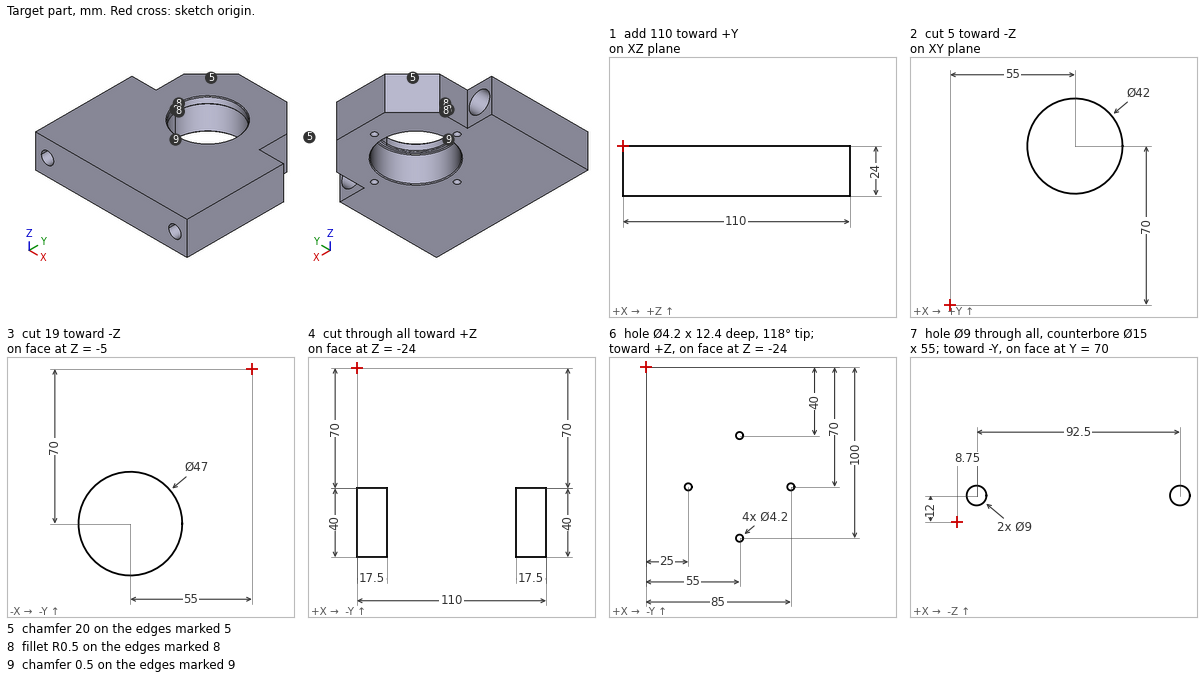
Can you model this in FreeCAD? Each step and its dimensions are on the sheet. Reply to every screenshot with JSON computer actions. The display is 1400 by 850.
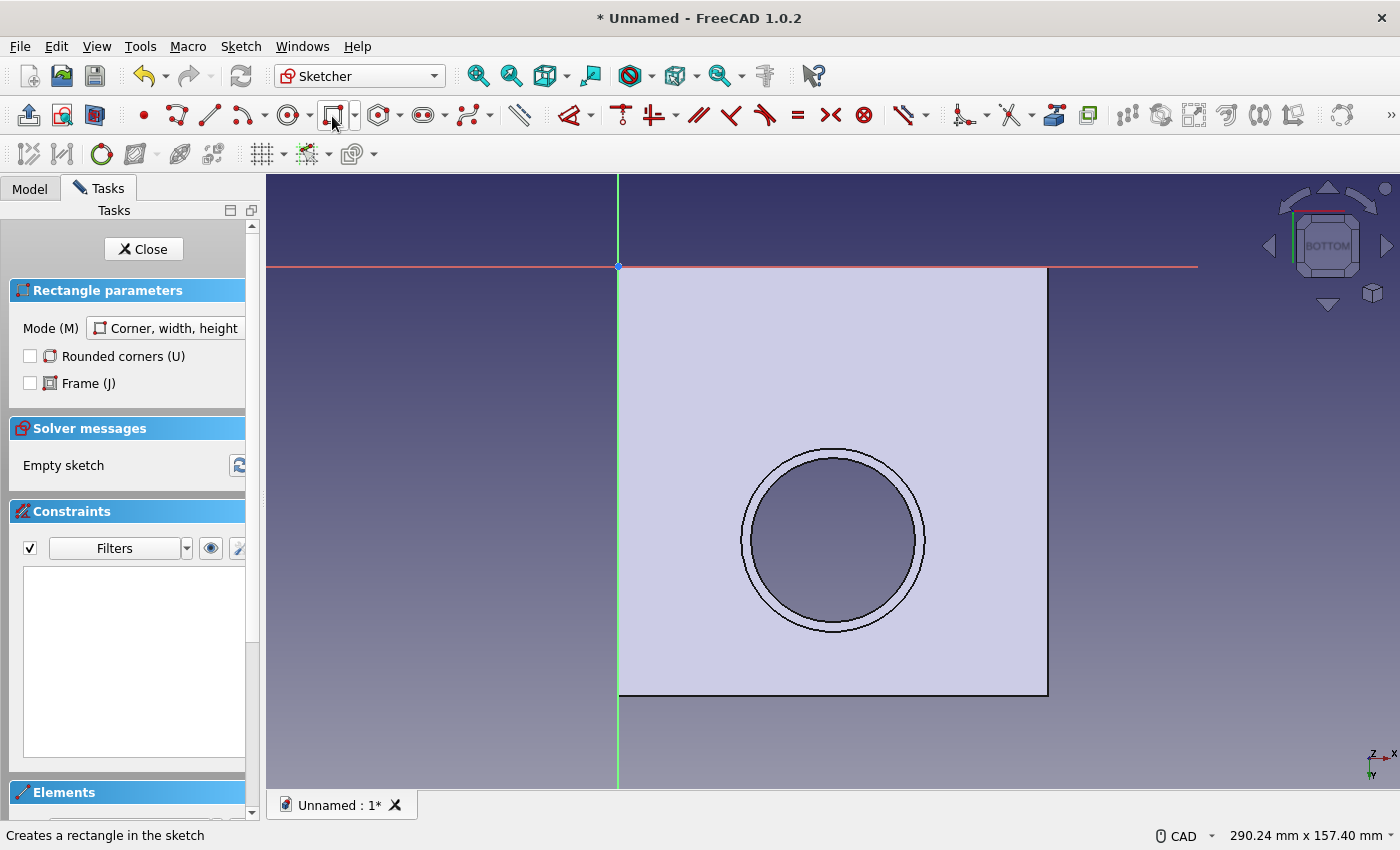
{"action": "left_click", "coordinate": [980, 540]}
{"action": "mouse_move", "coordinate": [1048, 696]}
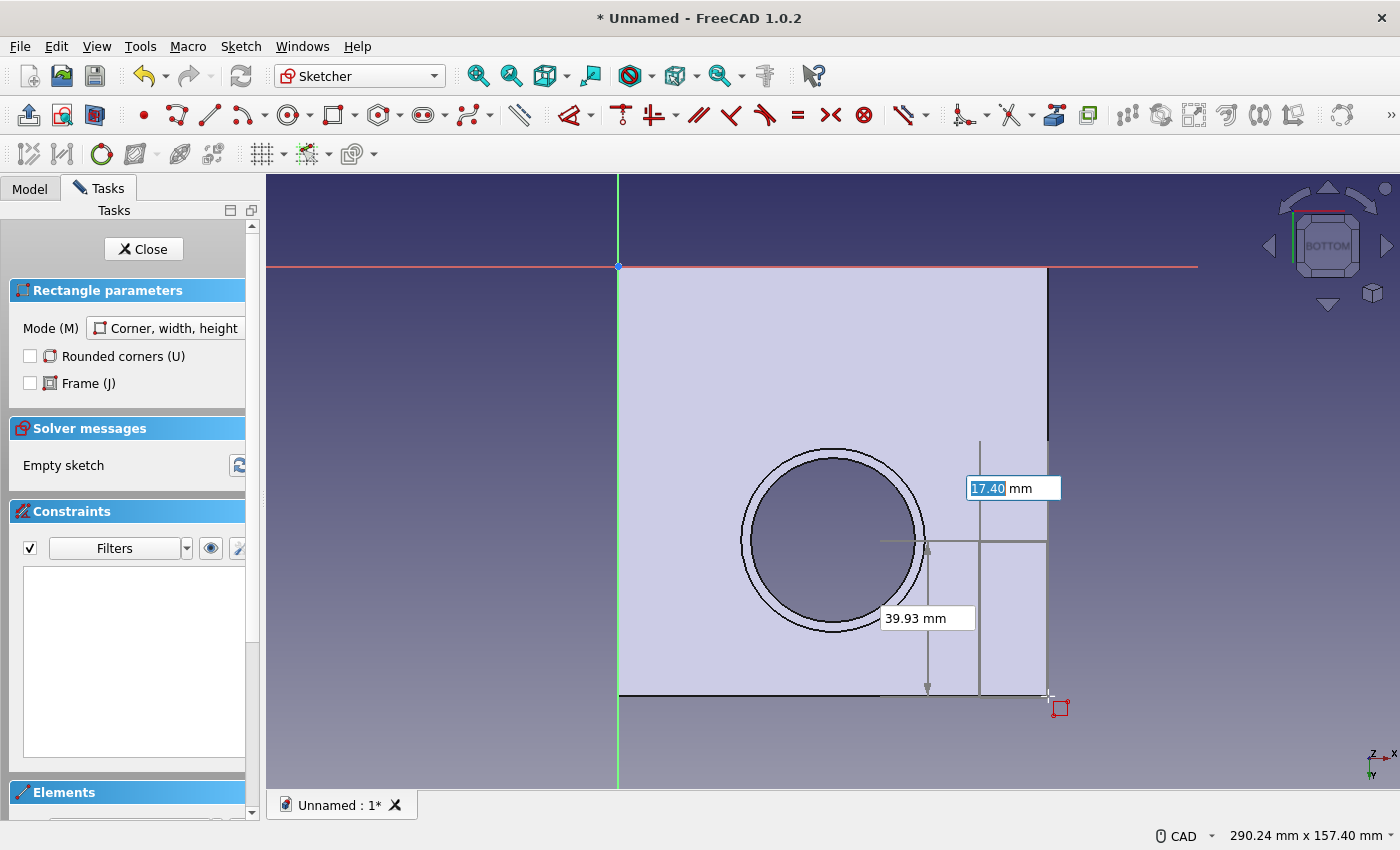
{"action": "type", "text": "17.5"}
{"action": "key", "text": "Tab"}
{"action": "type", "text": "40"}
{"action": "key", "text": "Return"}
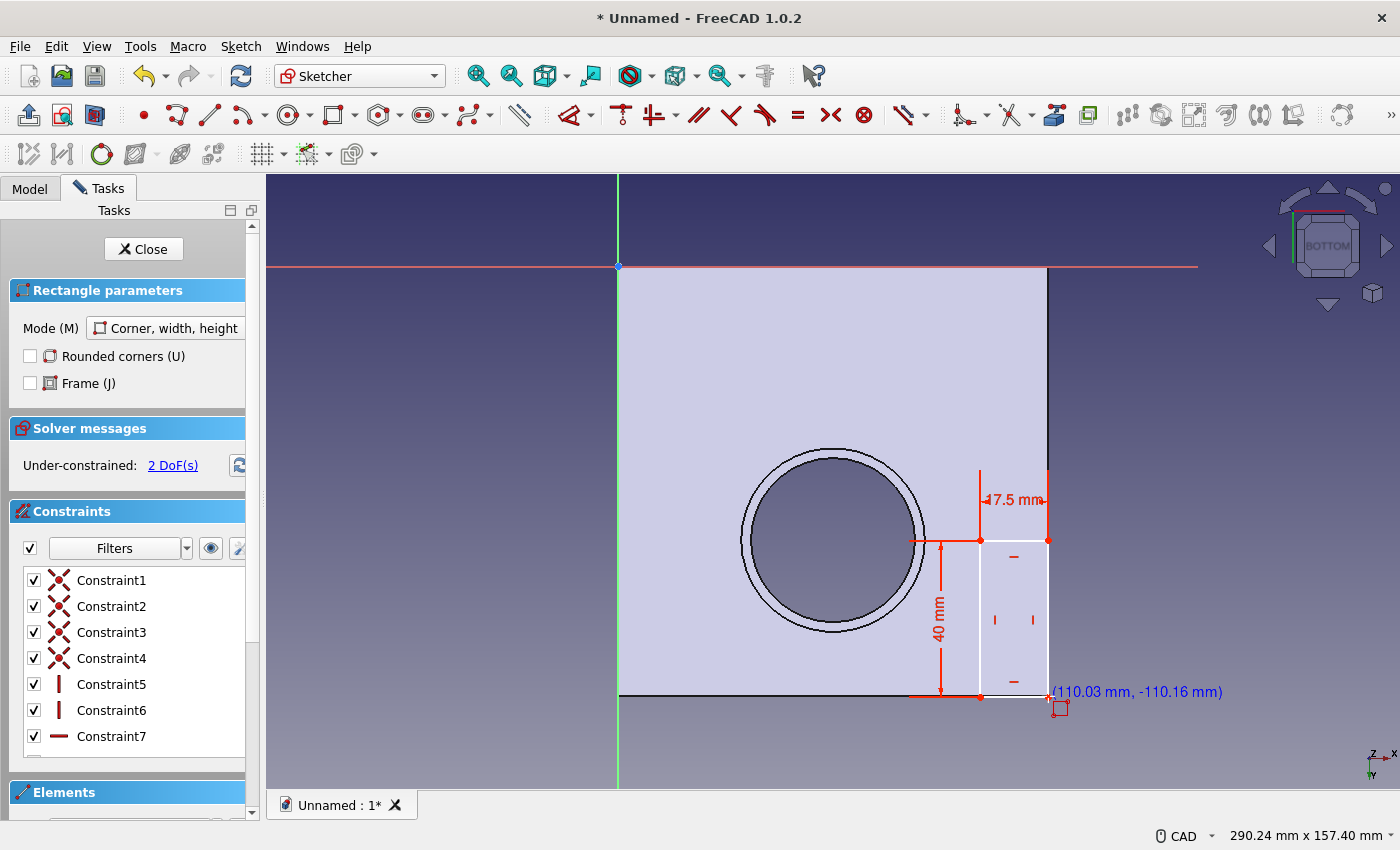
{"action": "left_click", "coordinate": [618, 540]}
{"action": "mouse_move", "coordinate": [686, 696]}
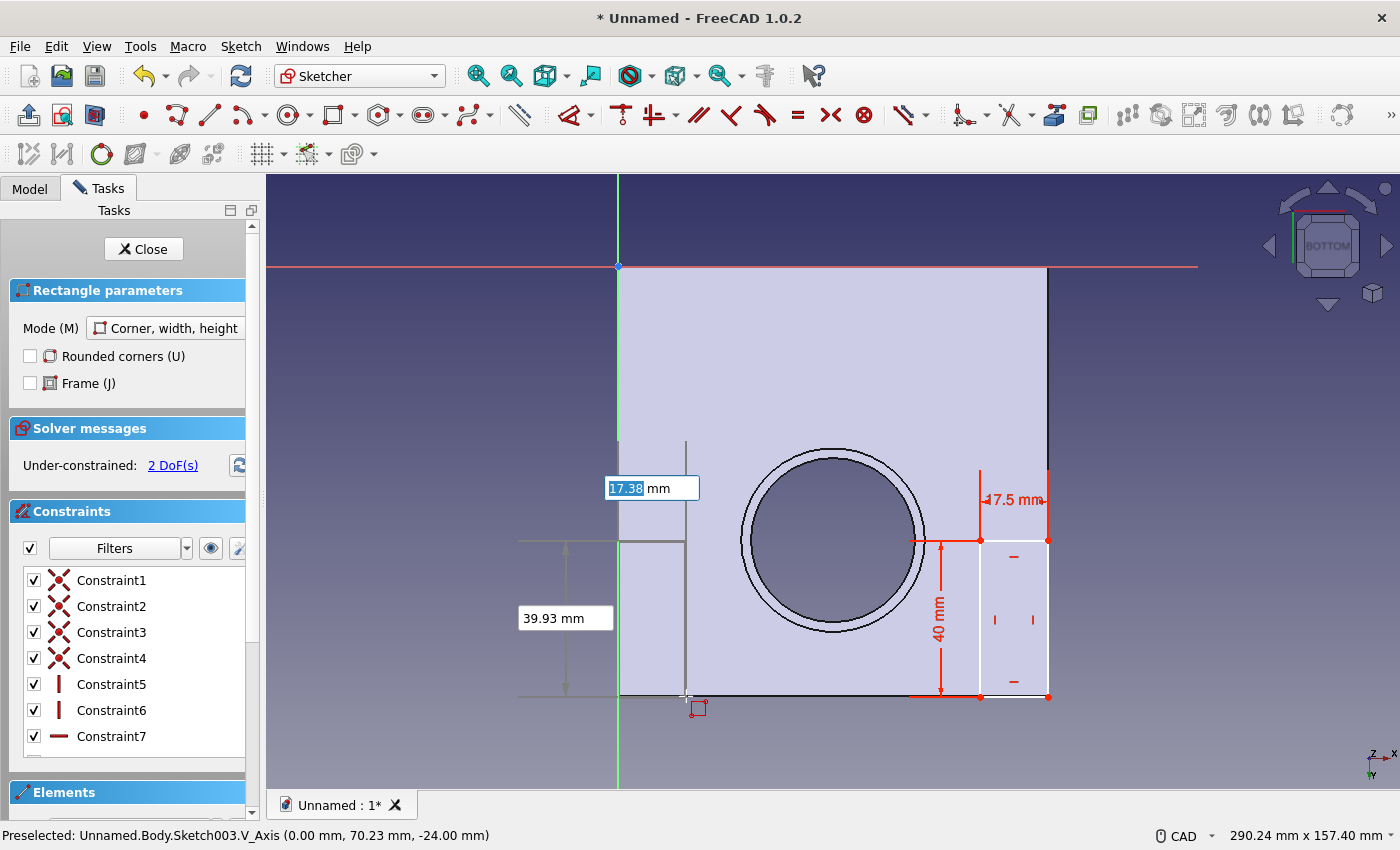
{"action": "type", "text": "17.5"}
{"action": "key", "text": "Tab"}
{"action": "type", "text": "40"}
{"action": "key", "text": "Return"}
{"action": "key", "text": "Escape"}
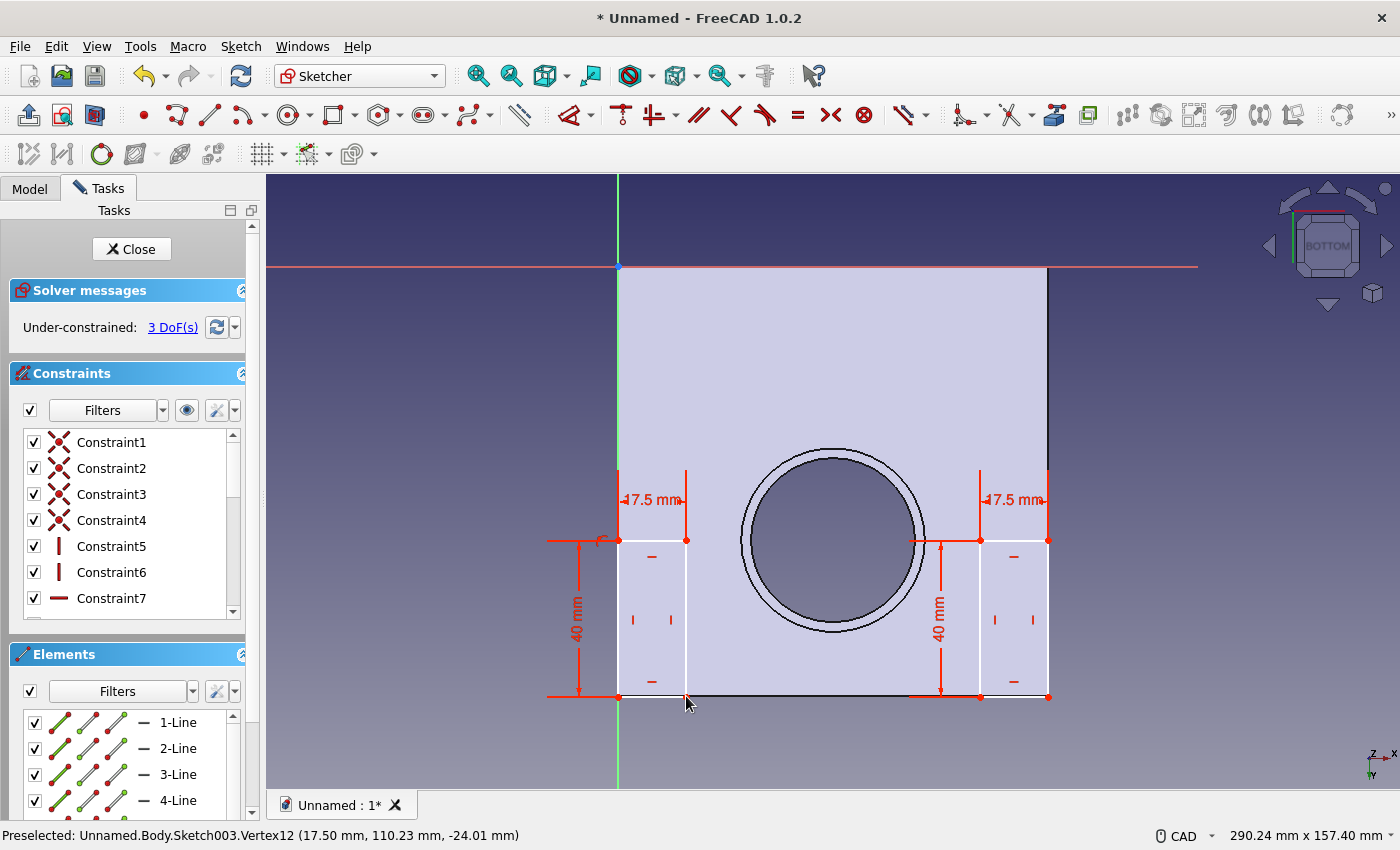
{"action": "left_click", "coordinate": [568, 116]}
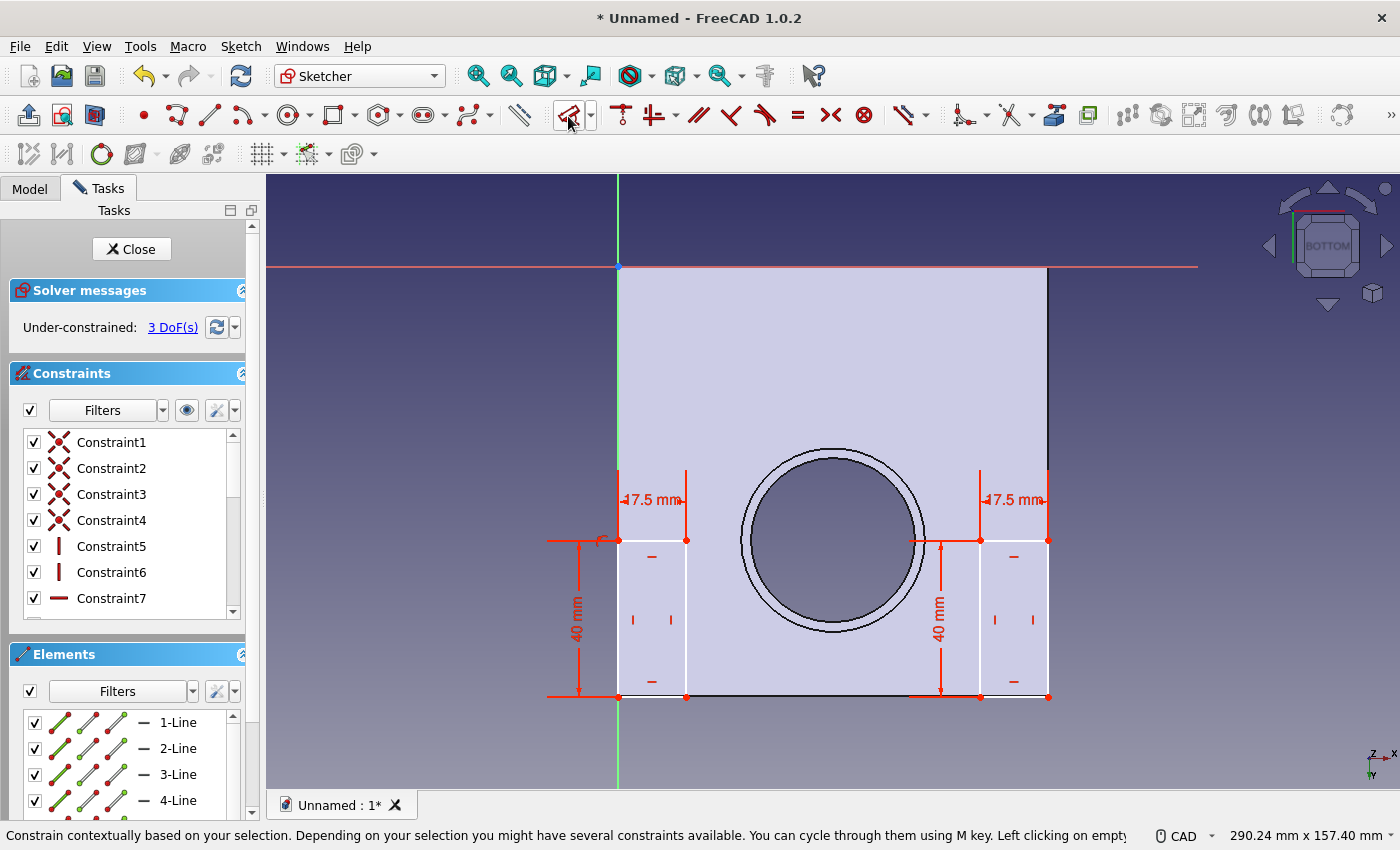
{"action": "left_click", "coordinate": [980, 541]}
{"action": "left_click", "coordinate": [584, 404]}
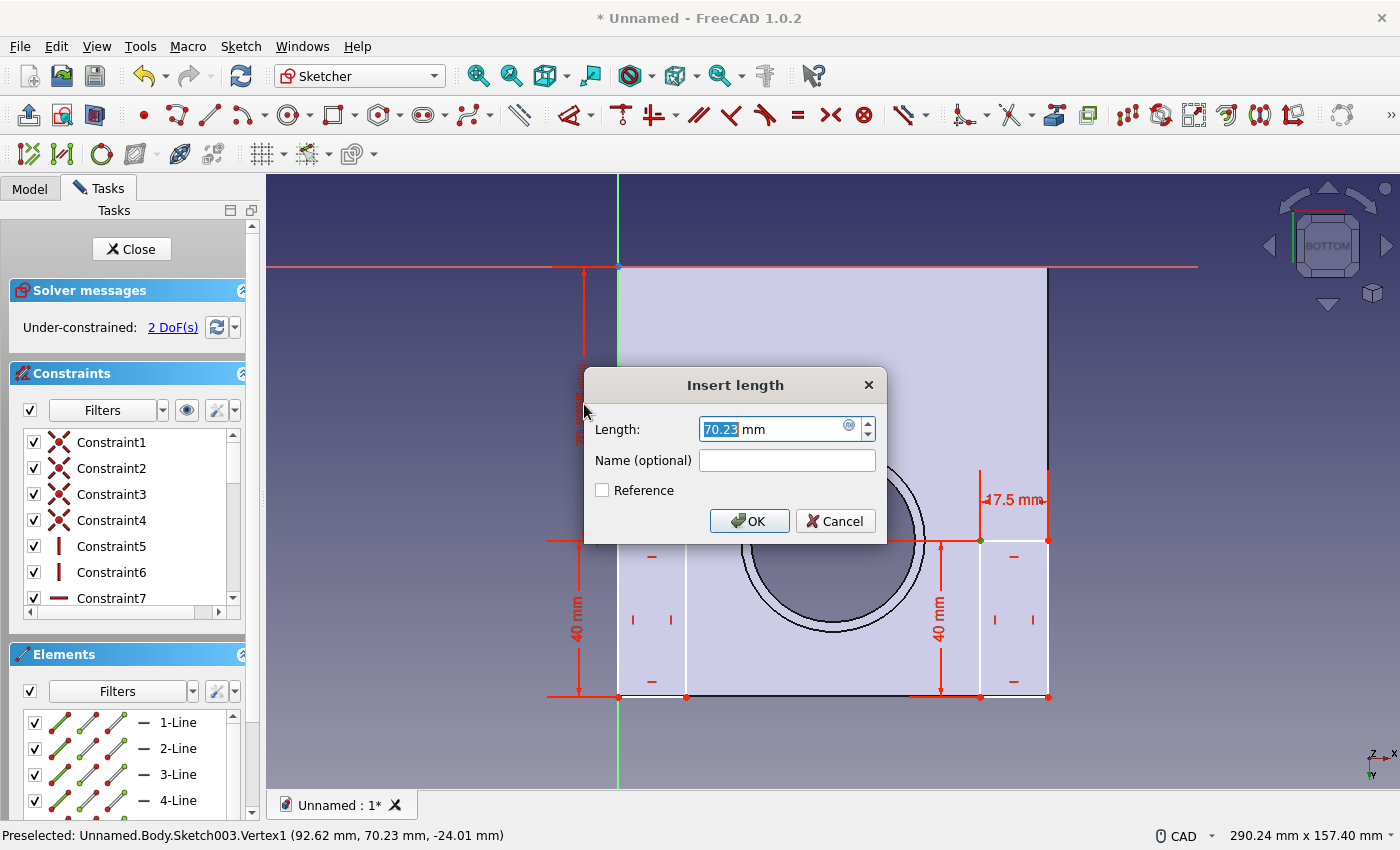
{"action": "type", "text": "70"}
{"action": "key", "text": "Return"}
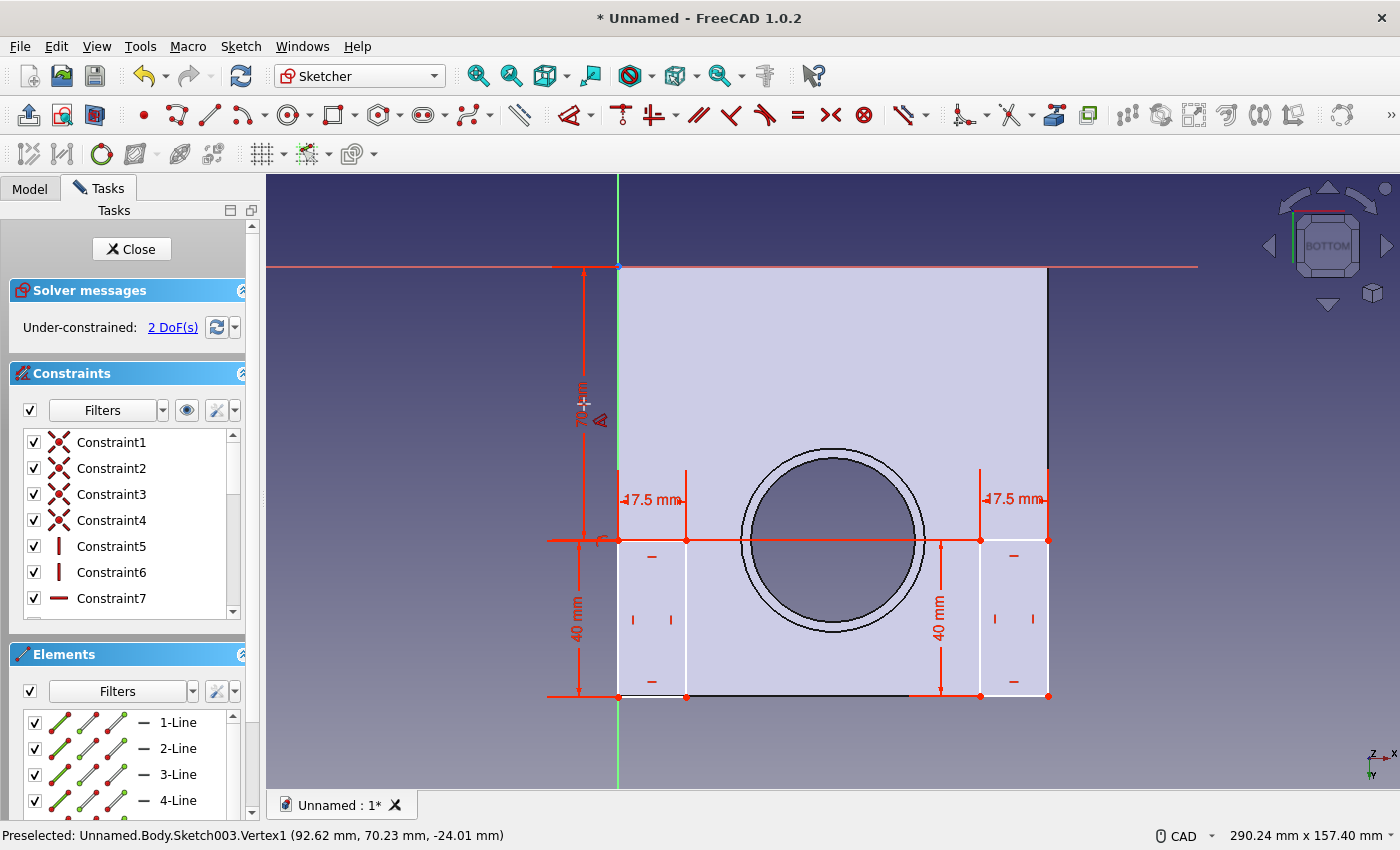
{"action": "left_click", "coordinate": [618, 541]}
{"action": "left_click", "coordinate": [584, 341]}